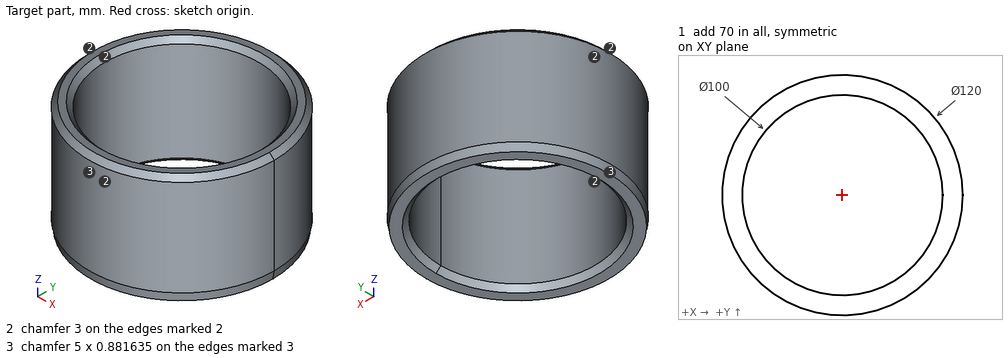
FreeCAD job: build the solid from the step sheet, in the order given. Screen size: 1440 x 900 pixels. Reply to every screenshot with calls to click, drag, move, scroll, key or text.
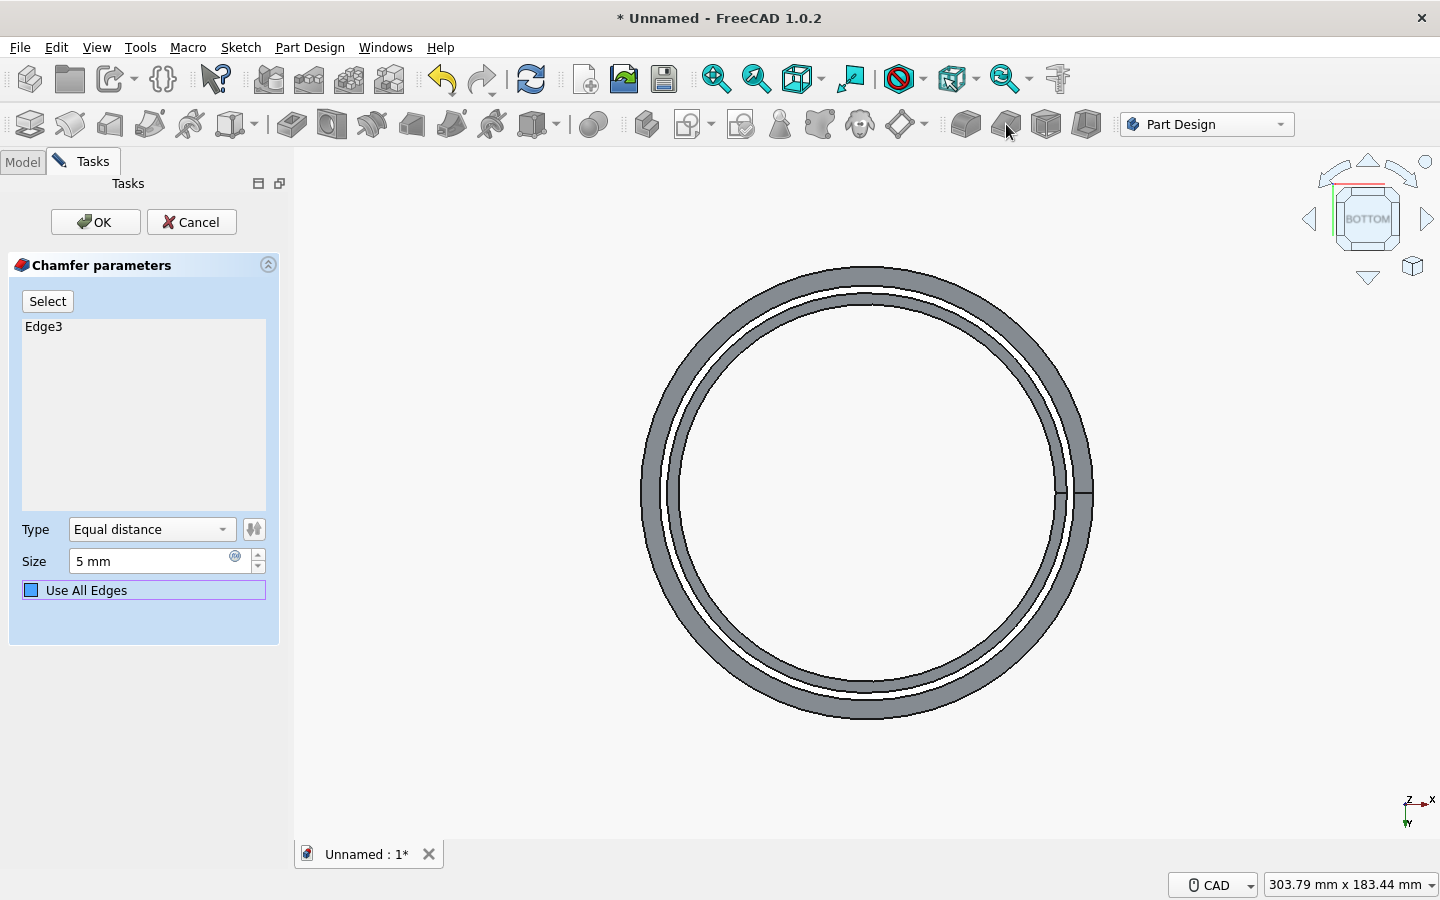
click(153, 530)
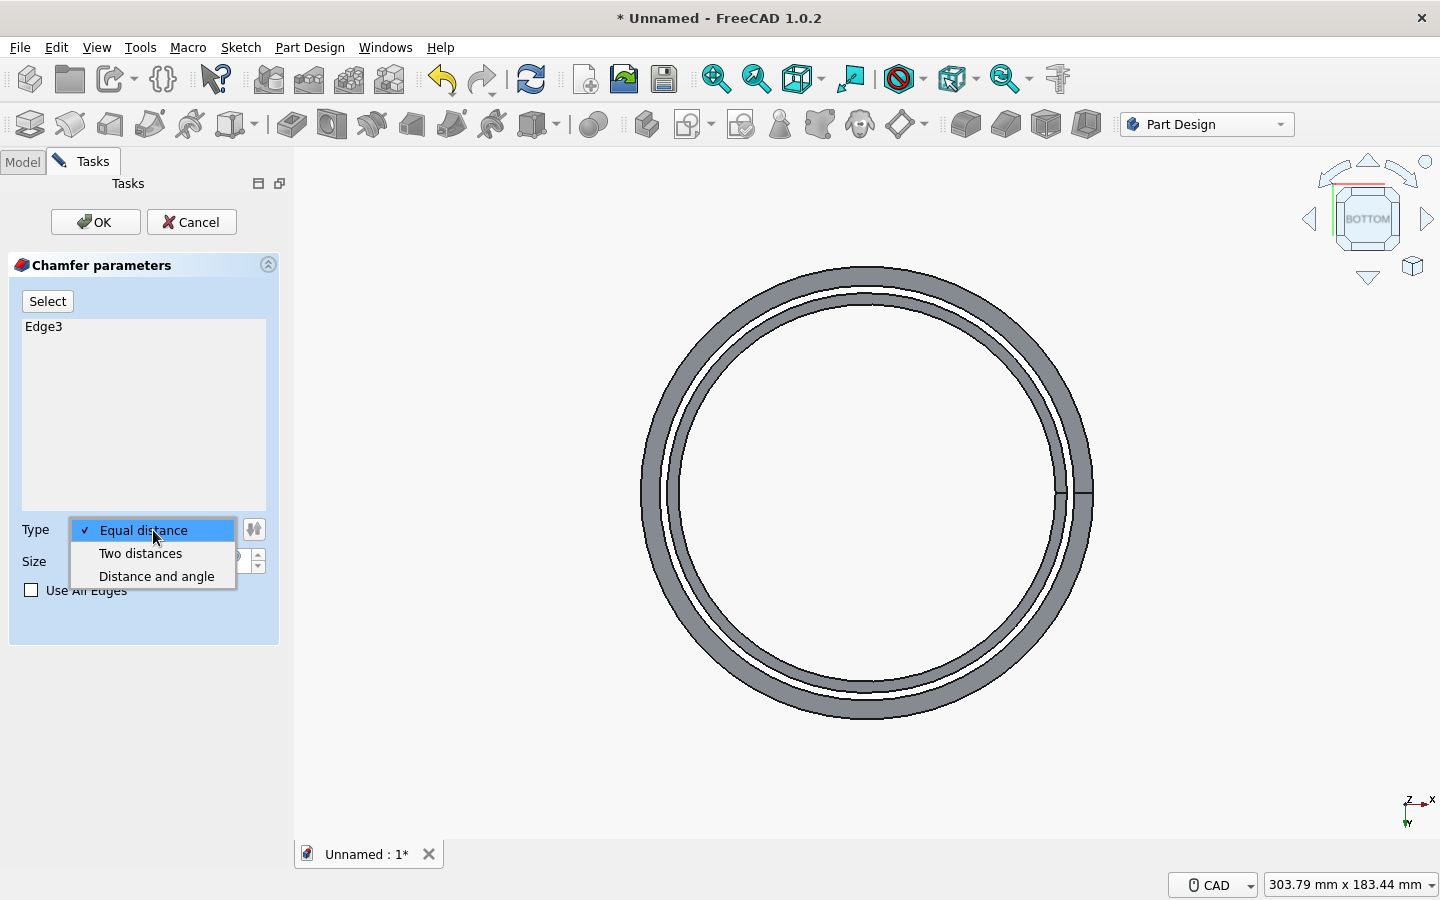
click(152, 554)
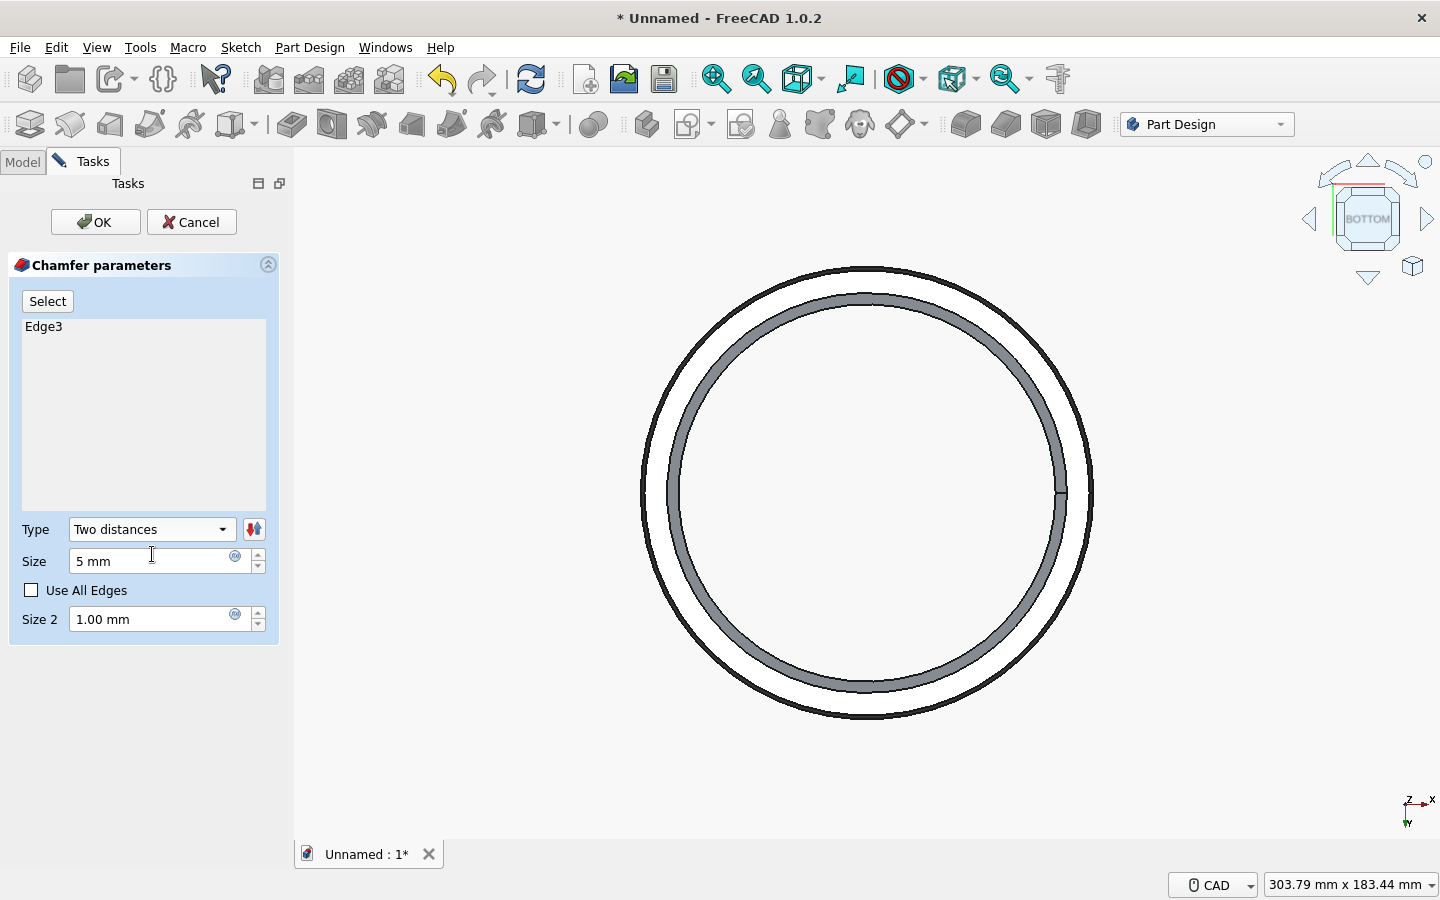
triple_click(160, 619)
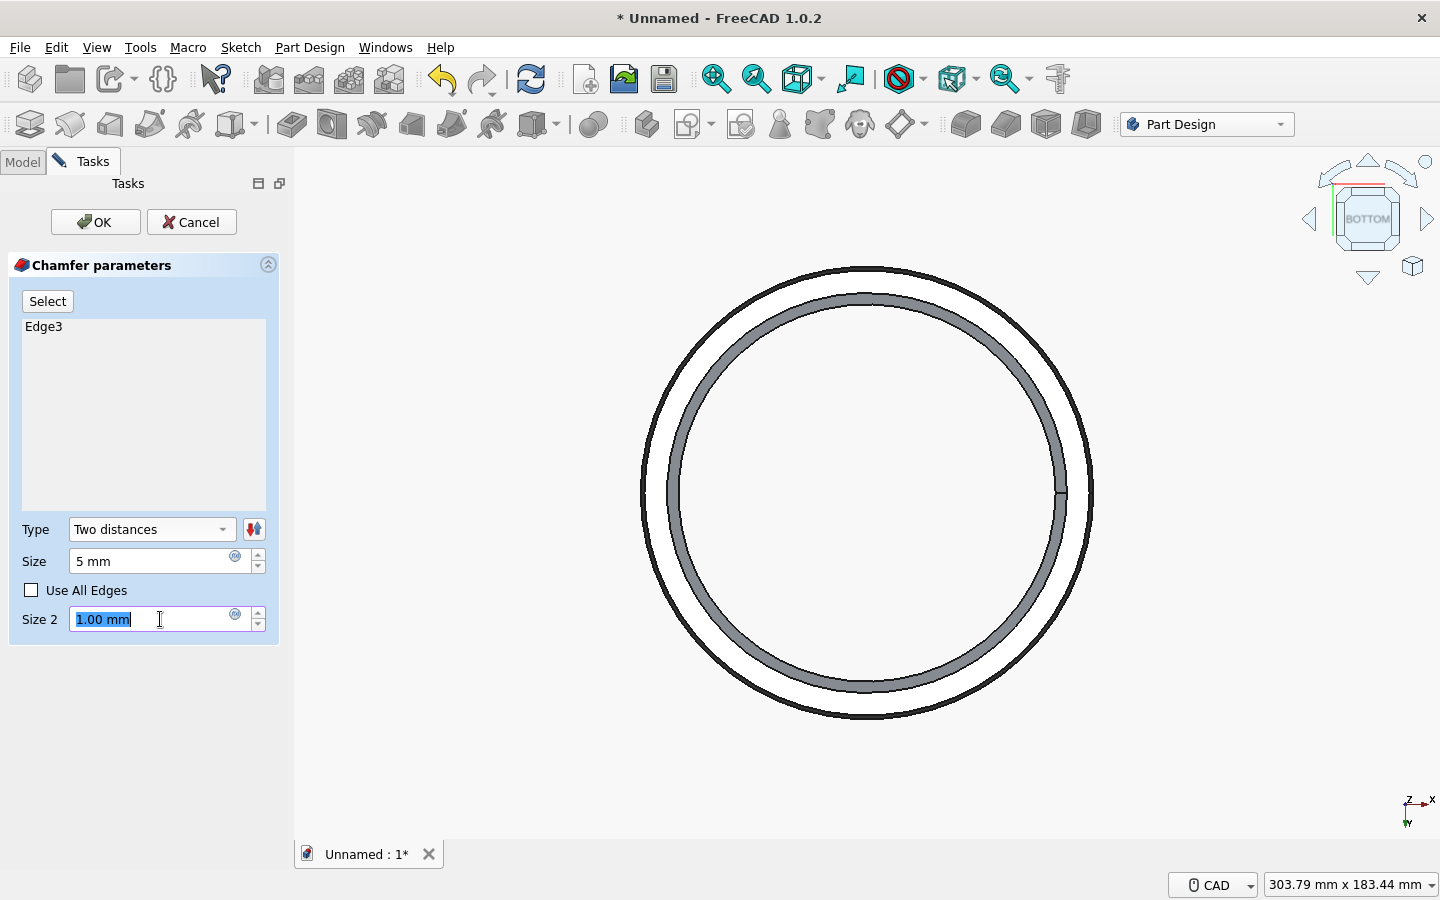
text(0.881635)
key(Tab)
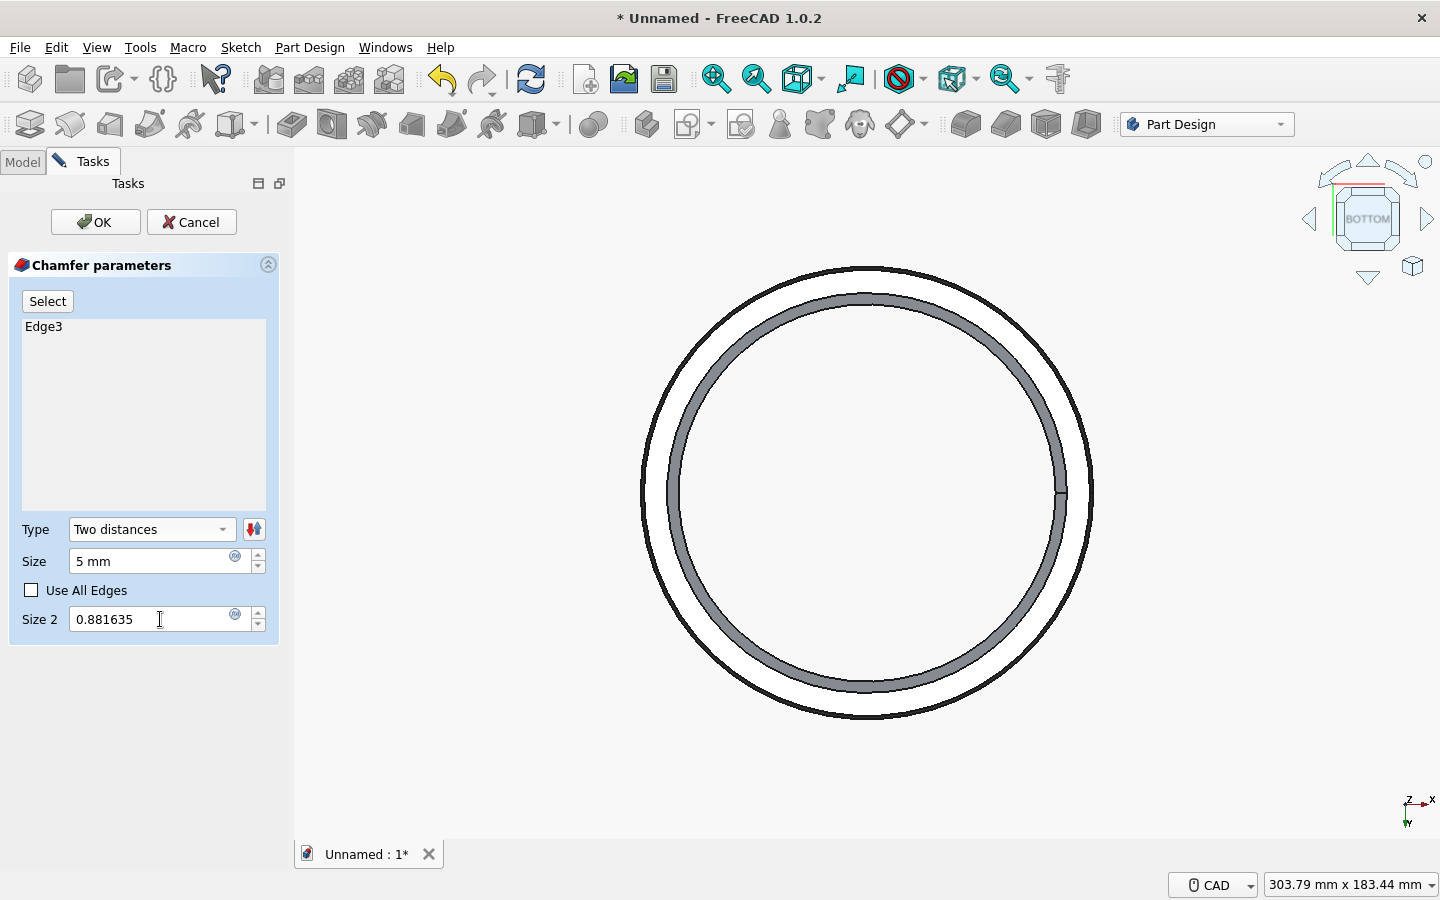
click(96, 222)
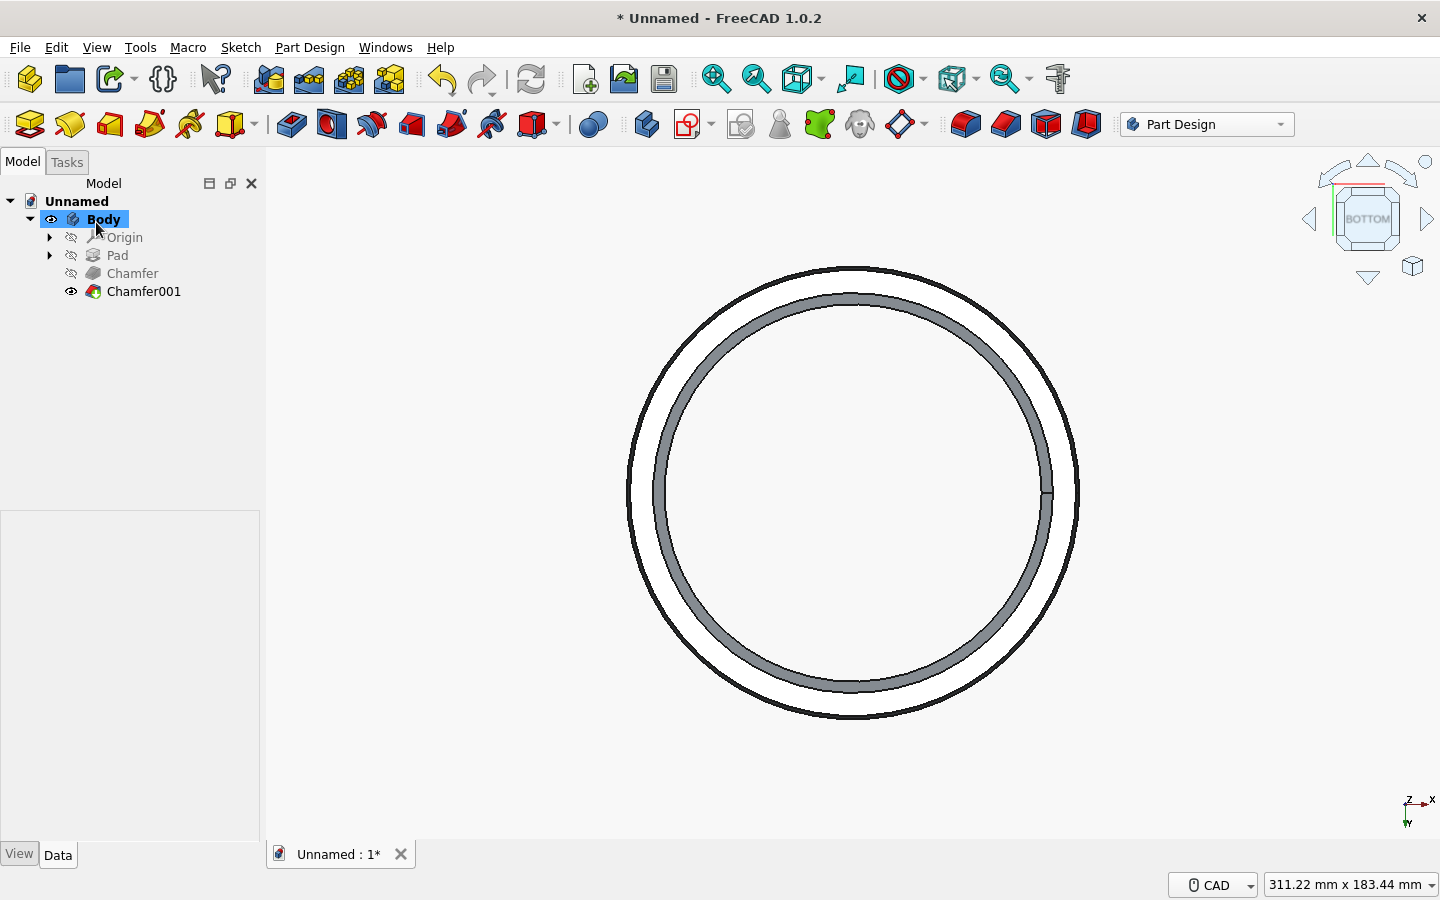
key(0)